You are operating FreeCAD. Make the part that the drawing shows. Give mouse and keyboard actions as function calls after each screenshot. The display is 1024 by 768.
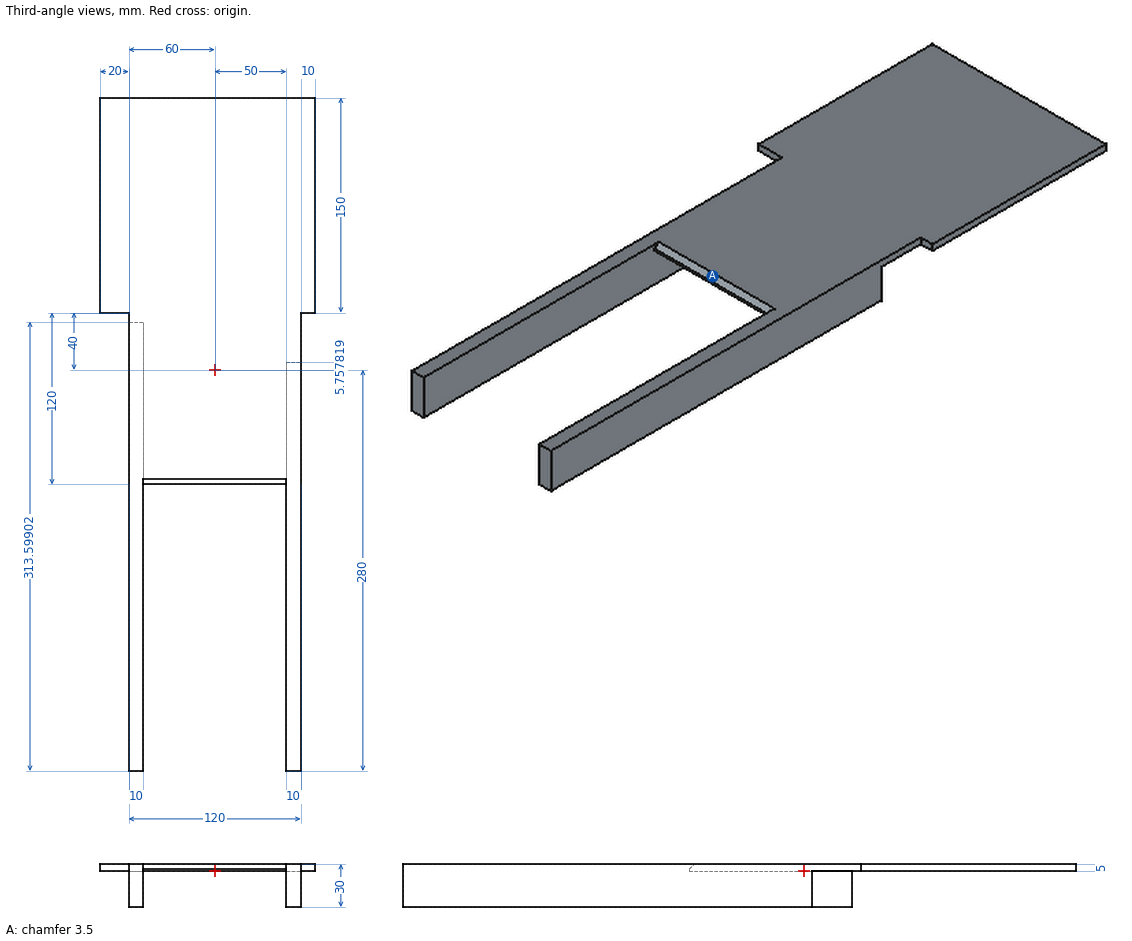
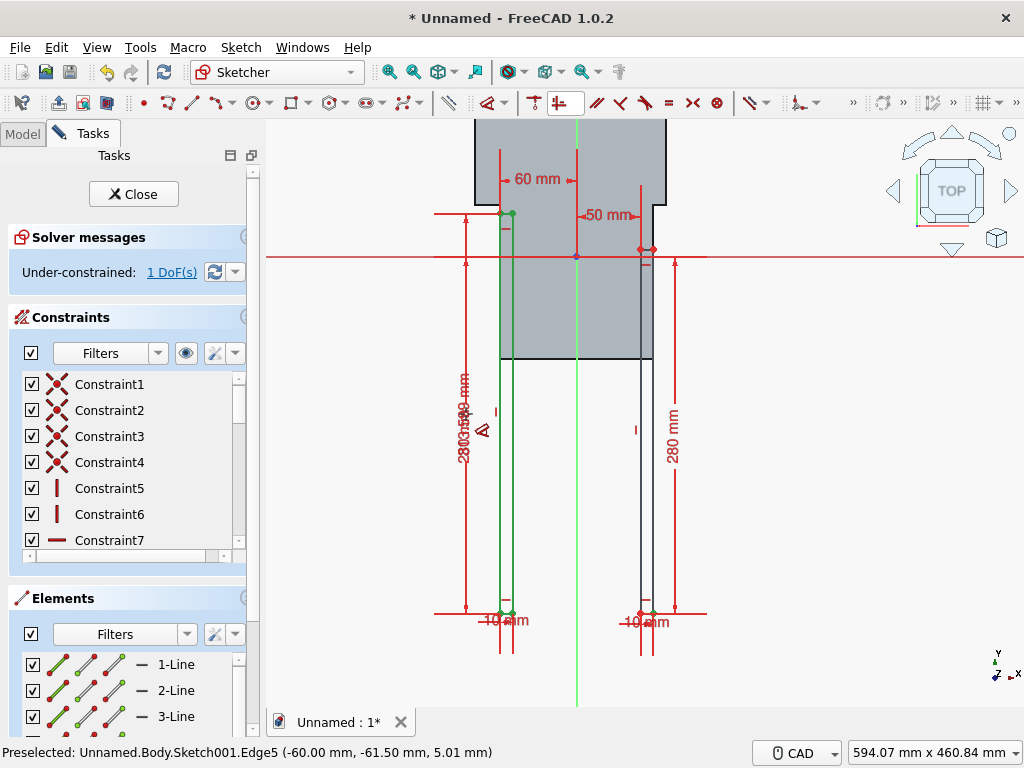
scroll(641, 250, up, 9)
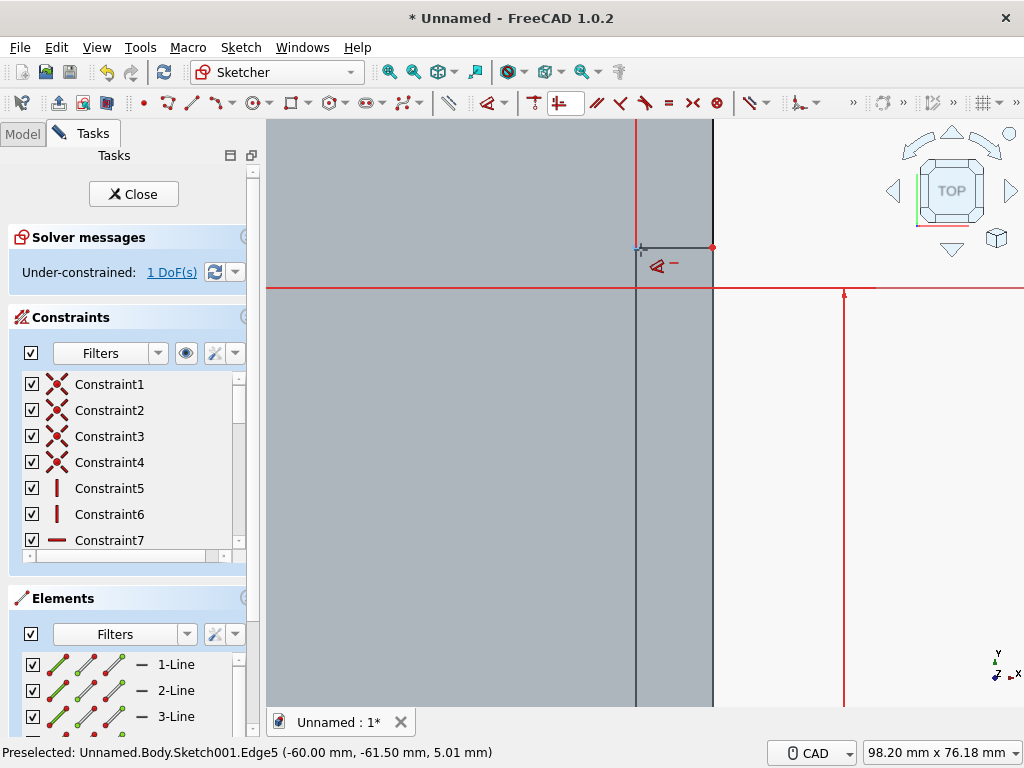
click(636, 248)
click(670, 268)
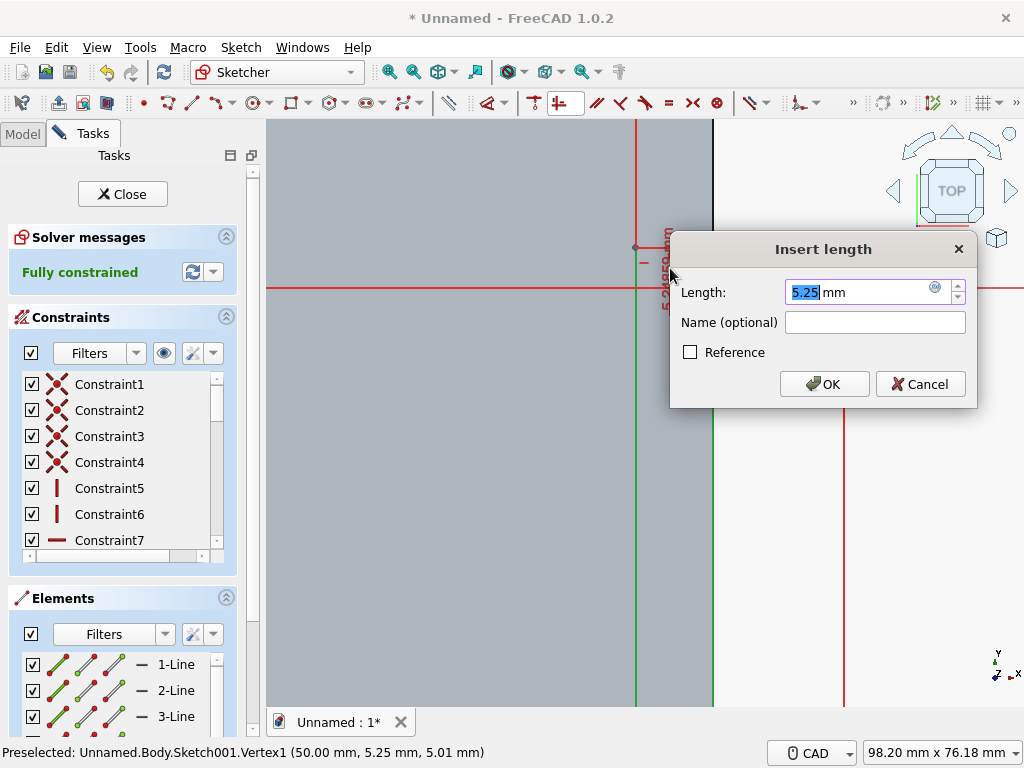
text(5.757819)
key(Return)
key(Escape)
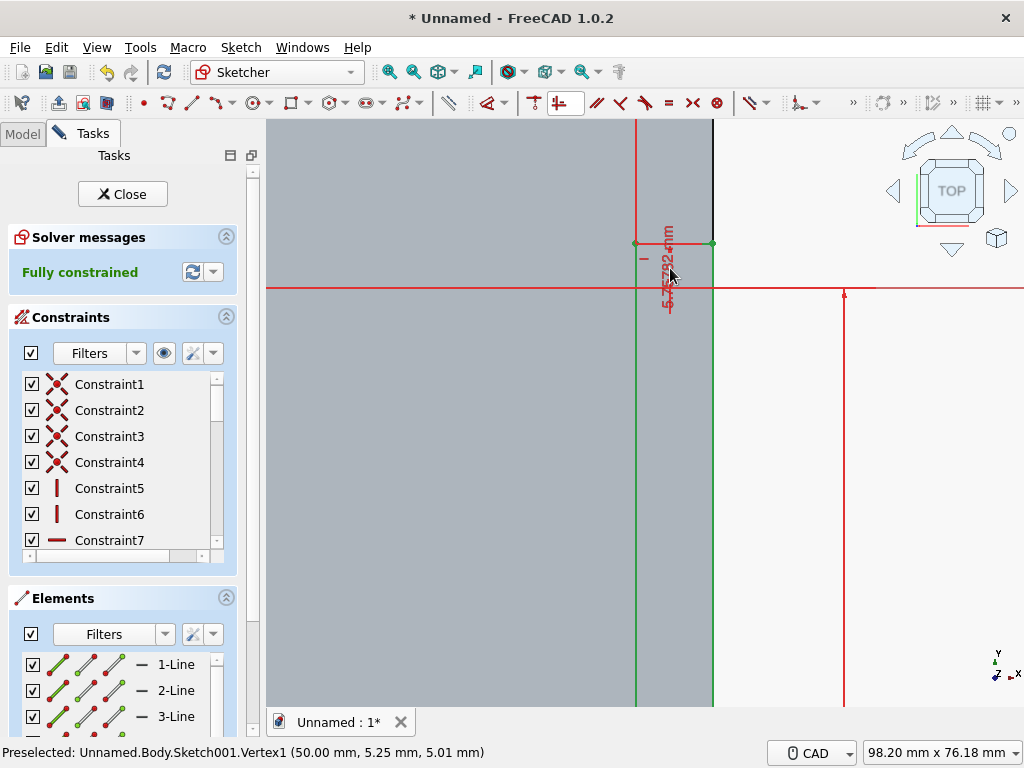
click(123, 194)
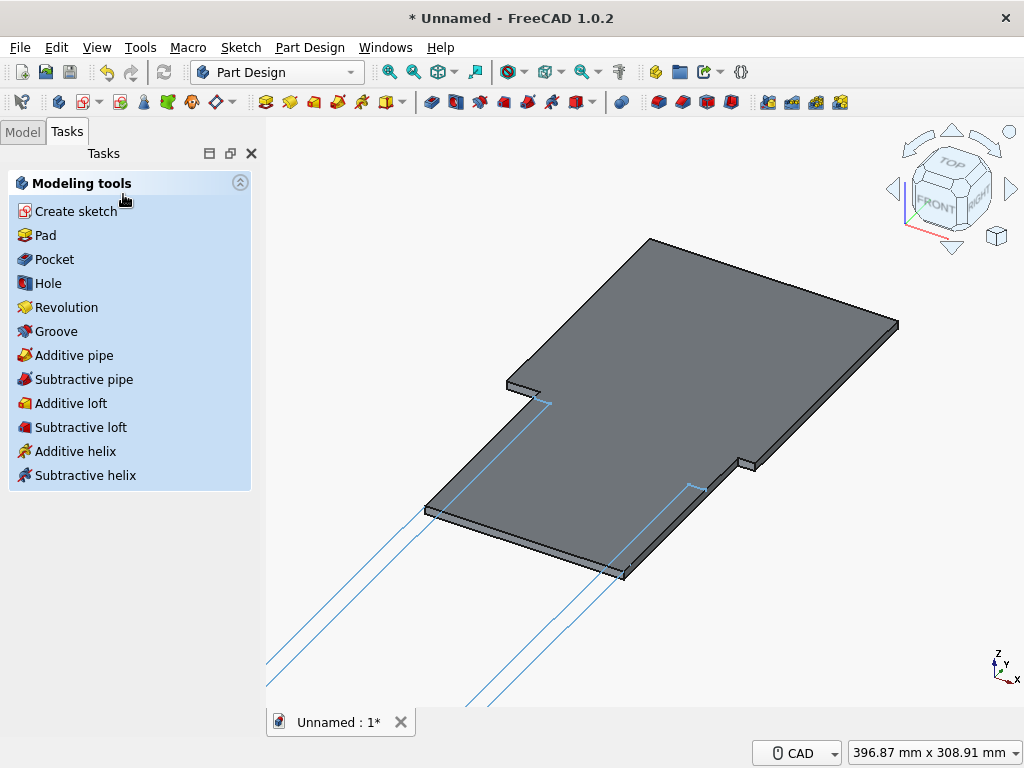
click(266, 102)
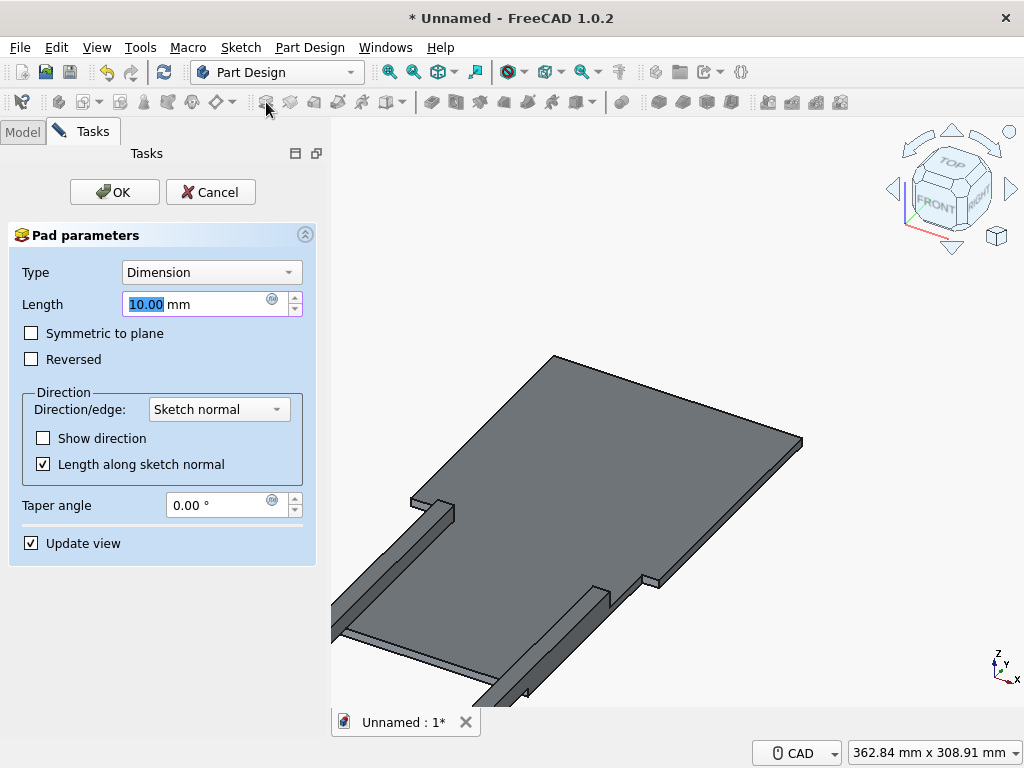
text(30)
key(Tab)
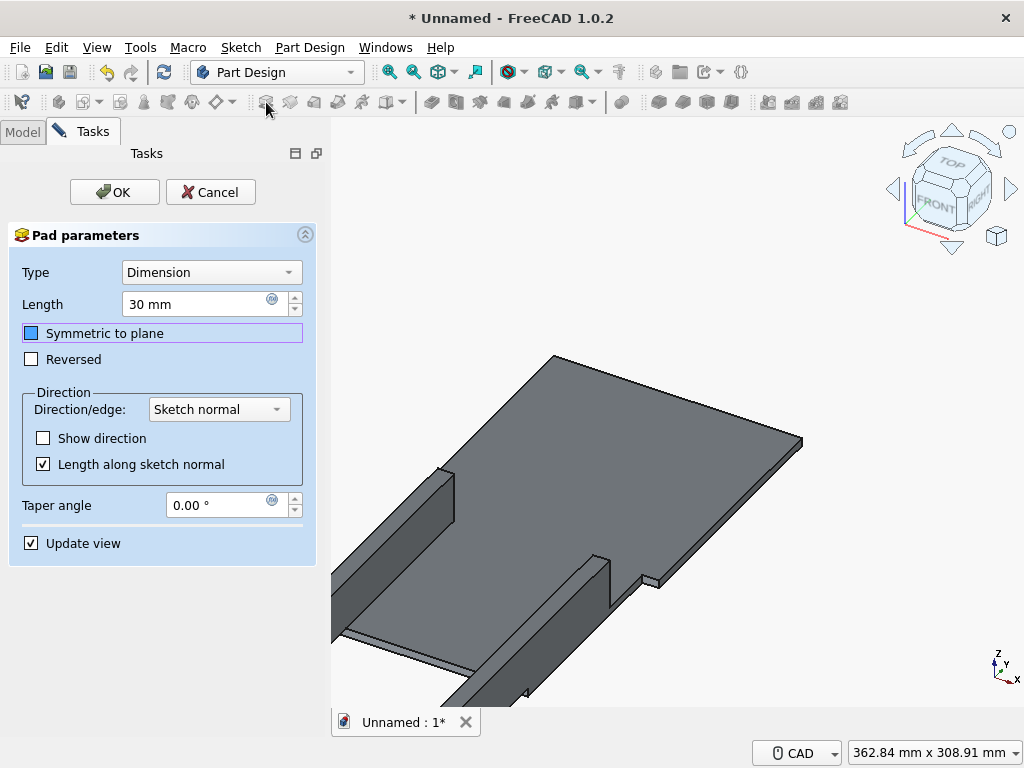
click(30, 359)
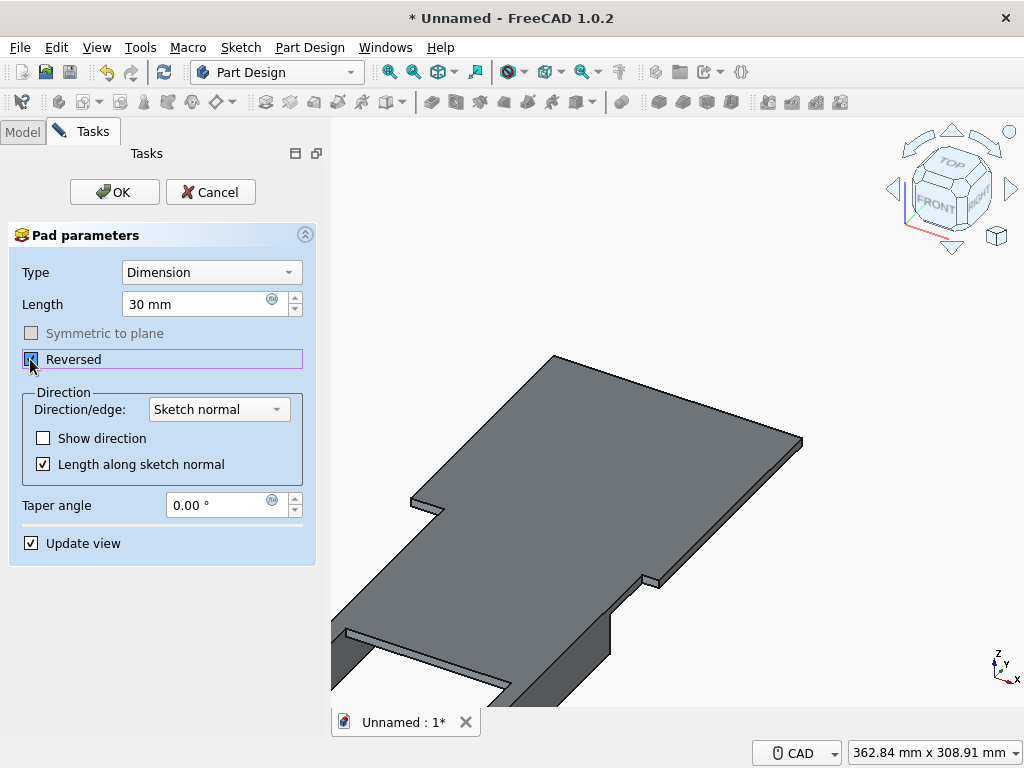
click(115, 192)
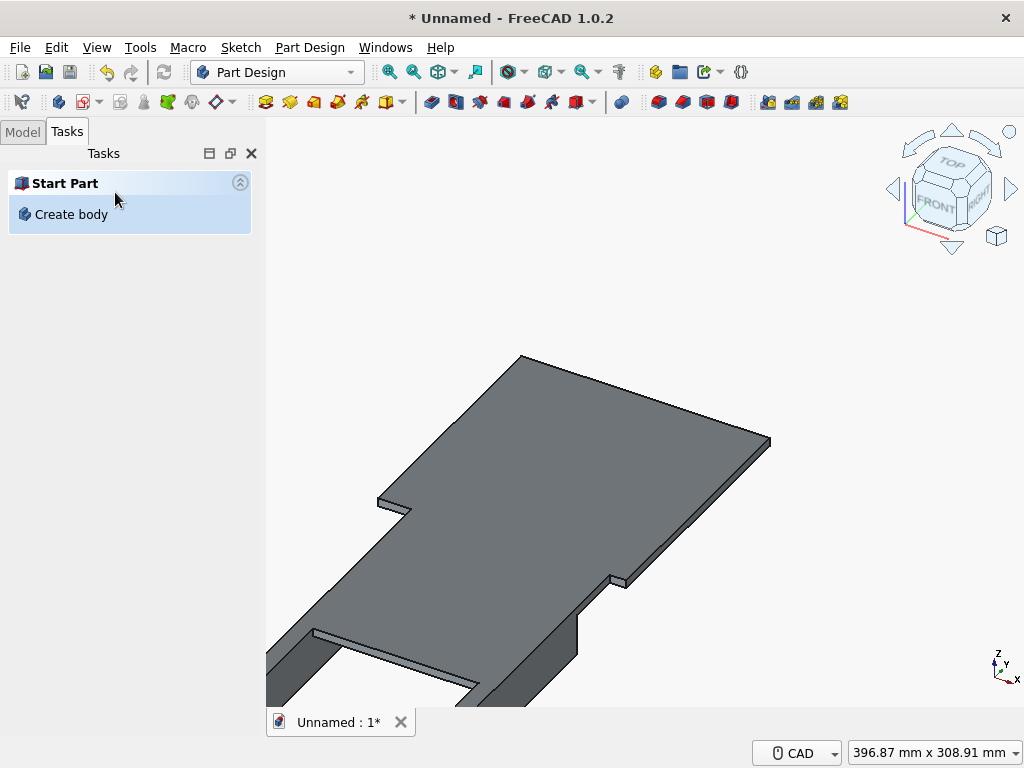
click(390, 72)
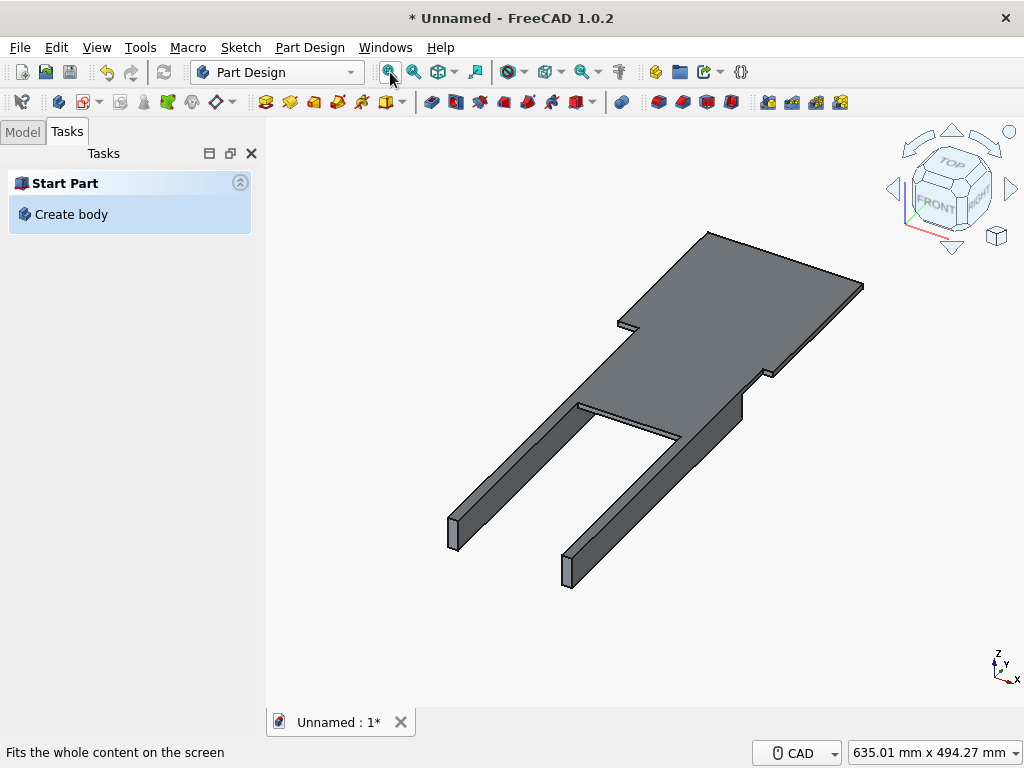
click(629, 419)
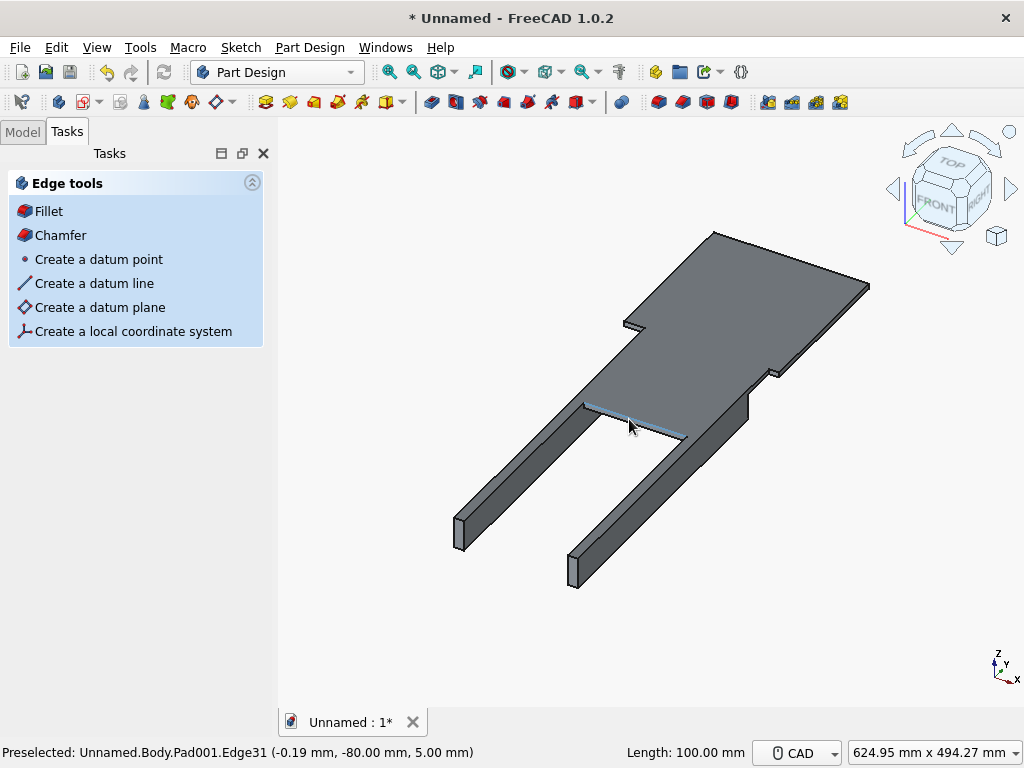
click(684, 102)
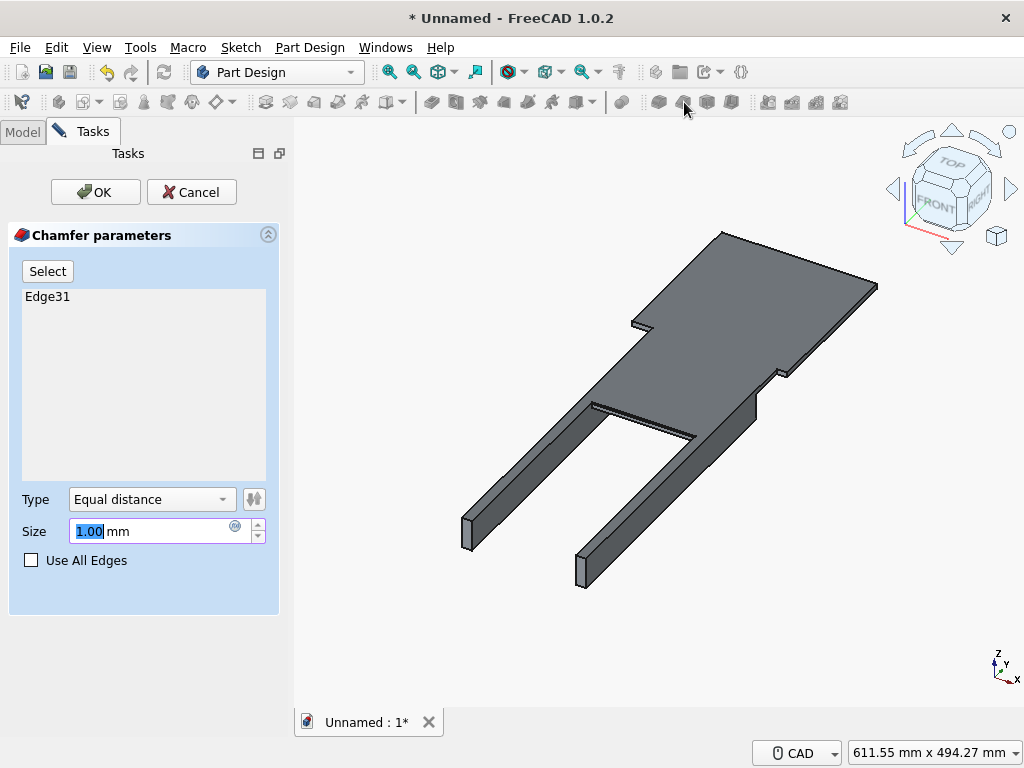
text(3.5)
key(Tab)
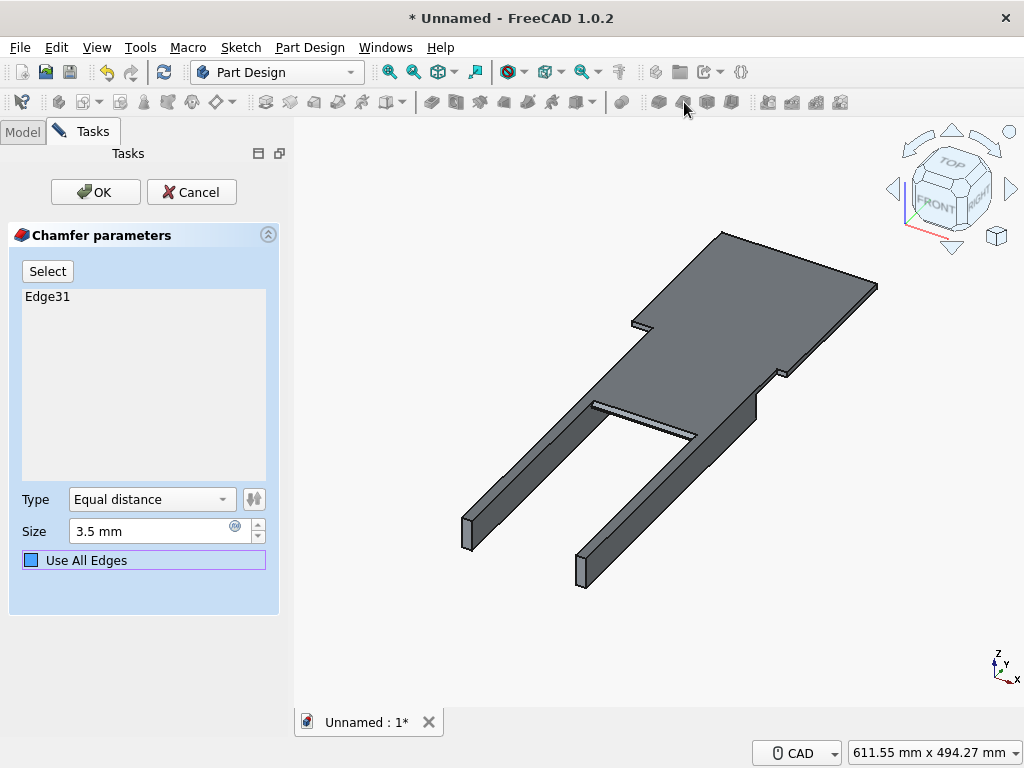
click(96, 192)